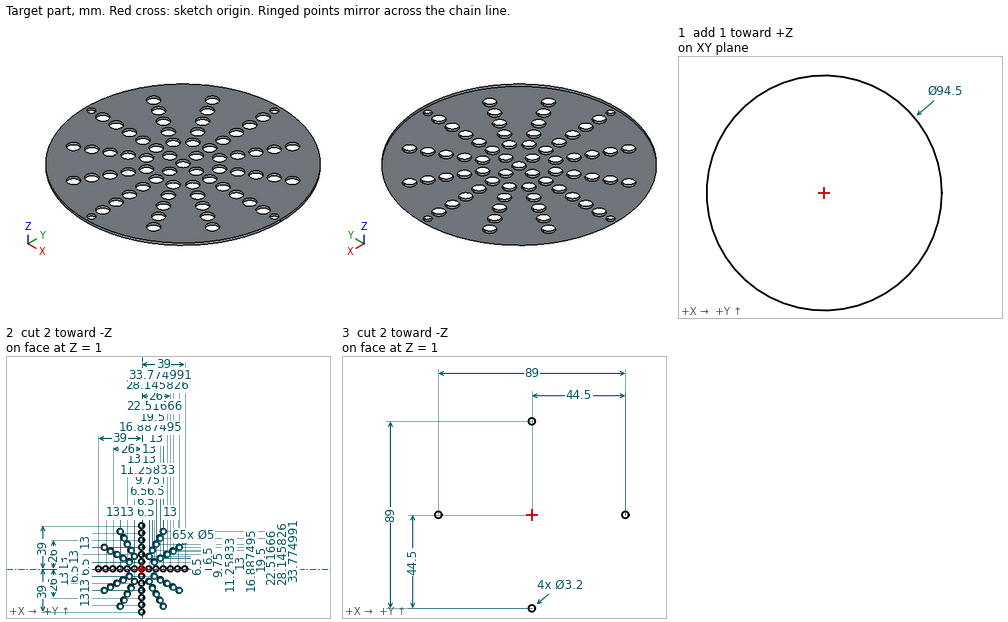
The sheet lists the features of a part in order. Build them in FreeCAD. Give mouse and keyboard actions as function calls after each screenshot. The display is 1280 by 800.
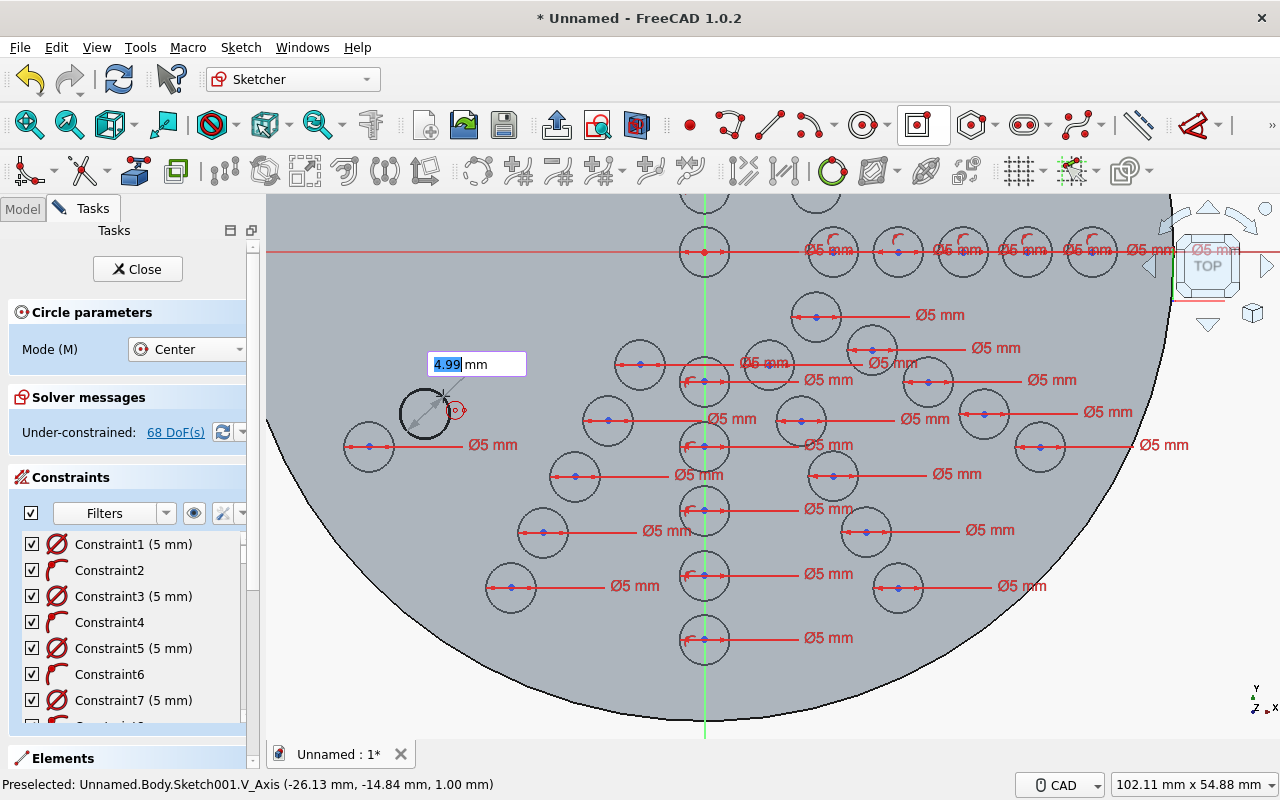
text(5)
key(Return)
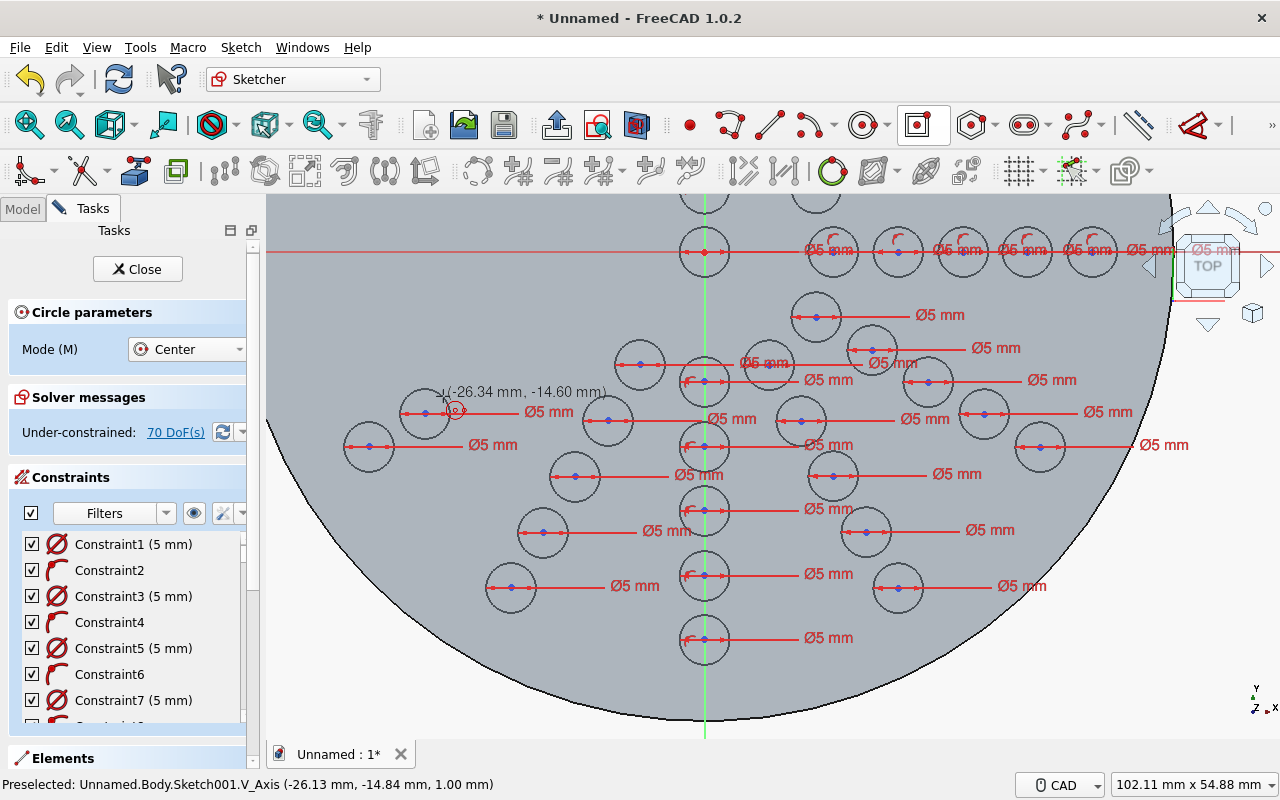
click(481, 381)
move(499, 364)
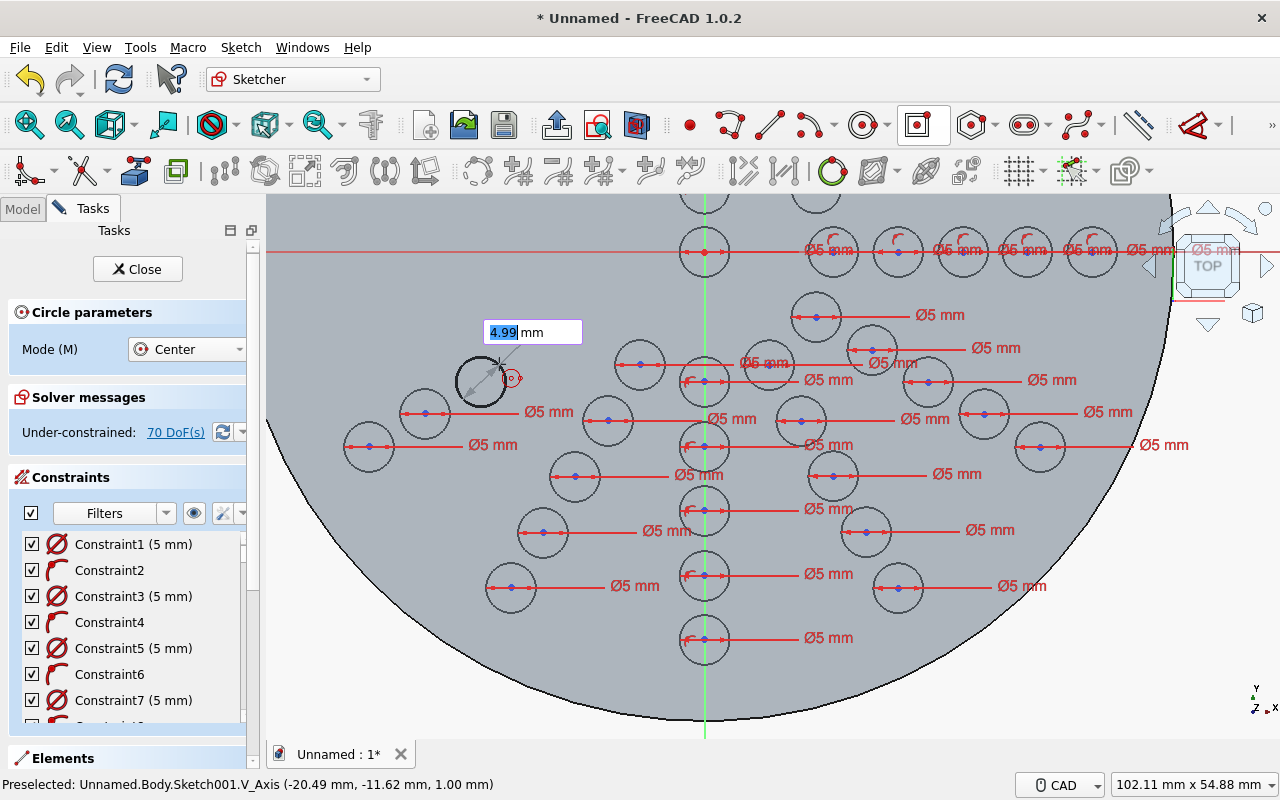
text(5)
key(Return)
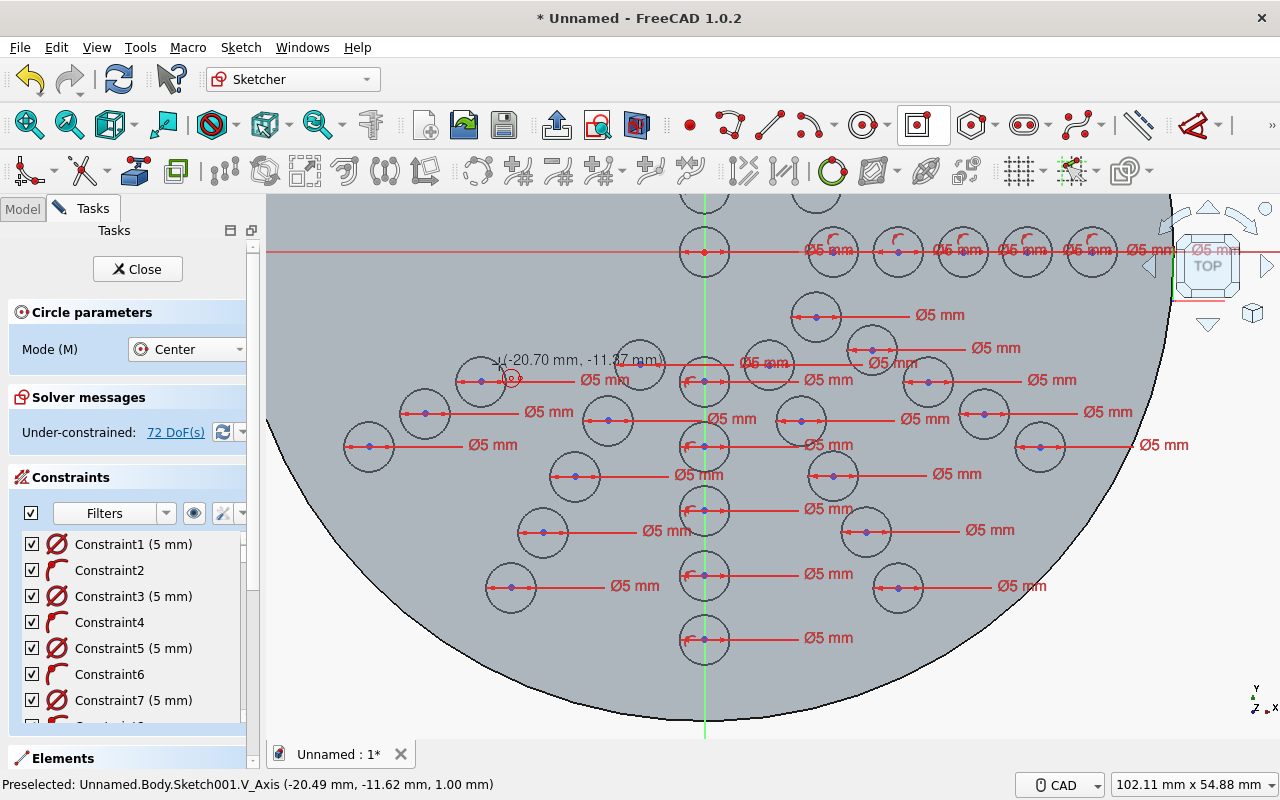
click(537, 349)
move(554, 331)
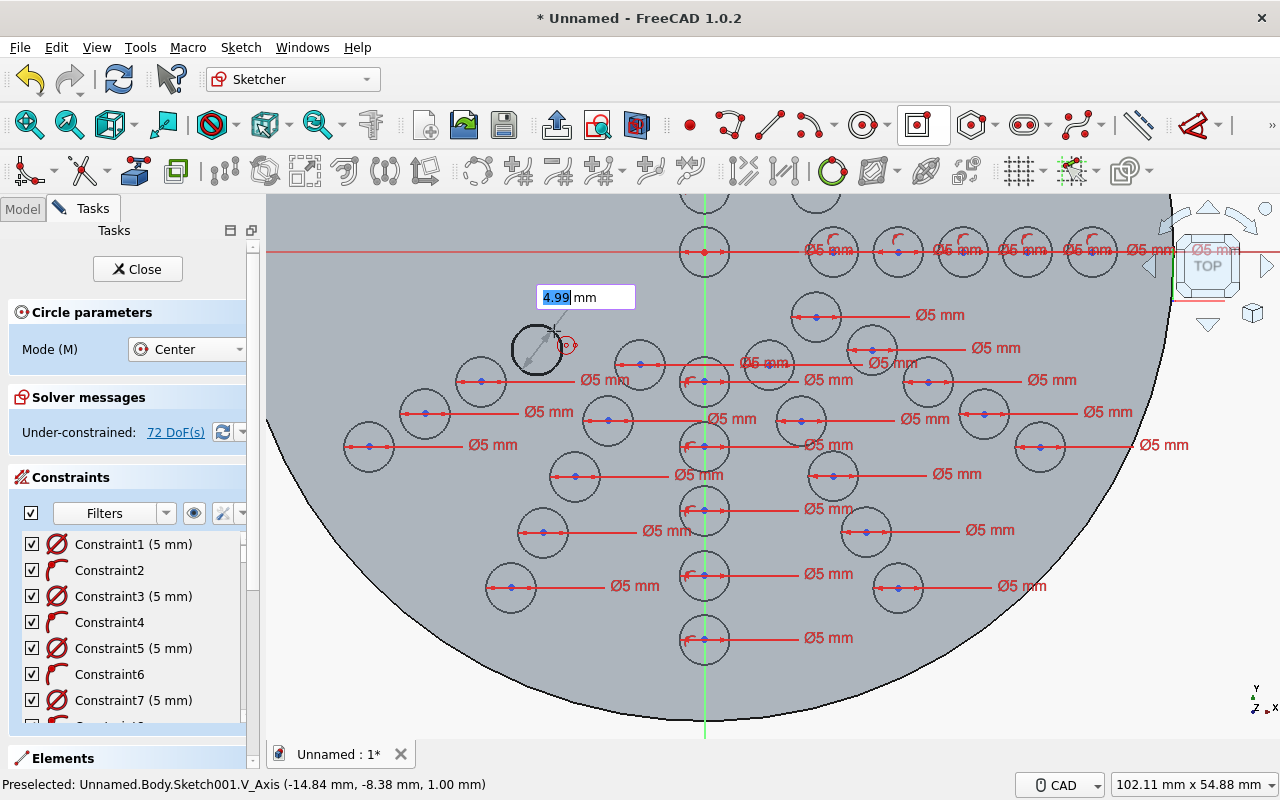
text(5)
key(Return)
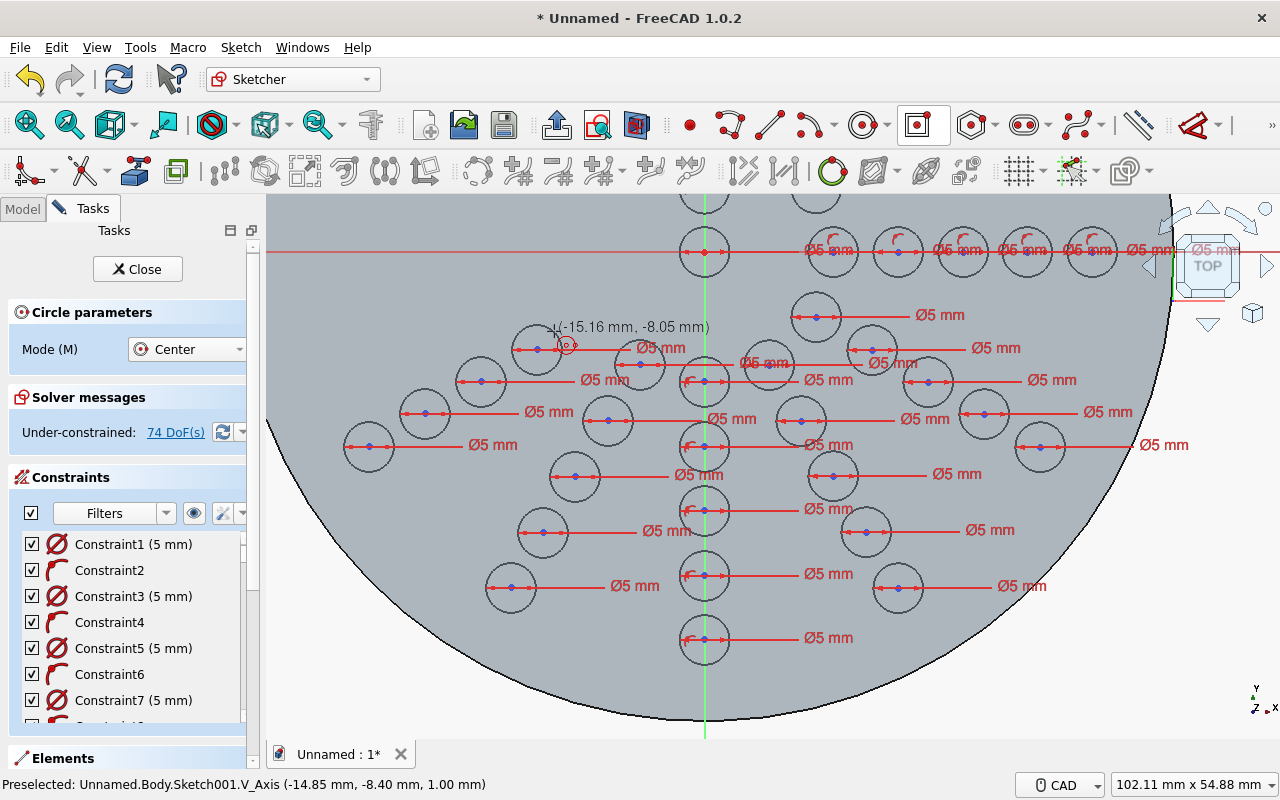
click(593, 317)
move(610, 299)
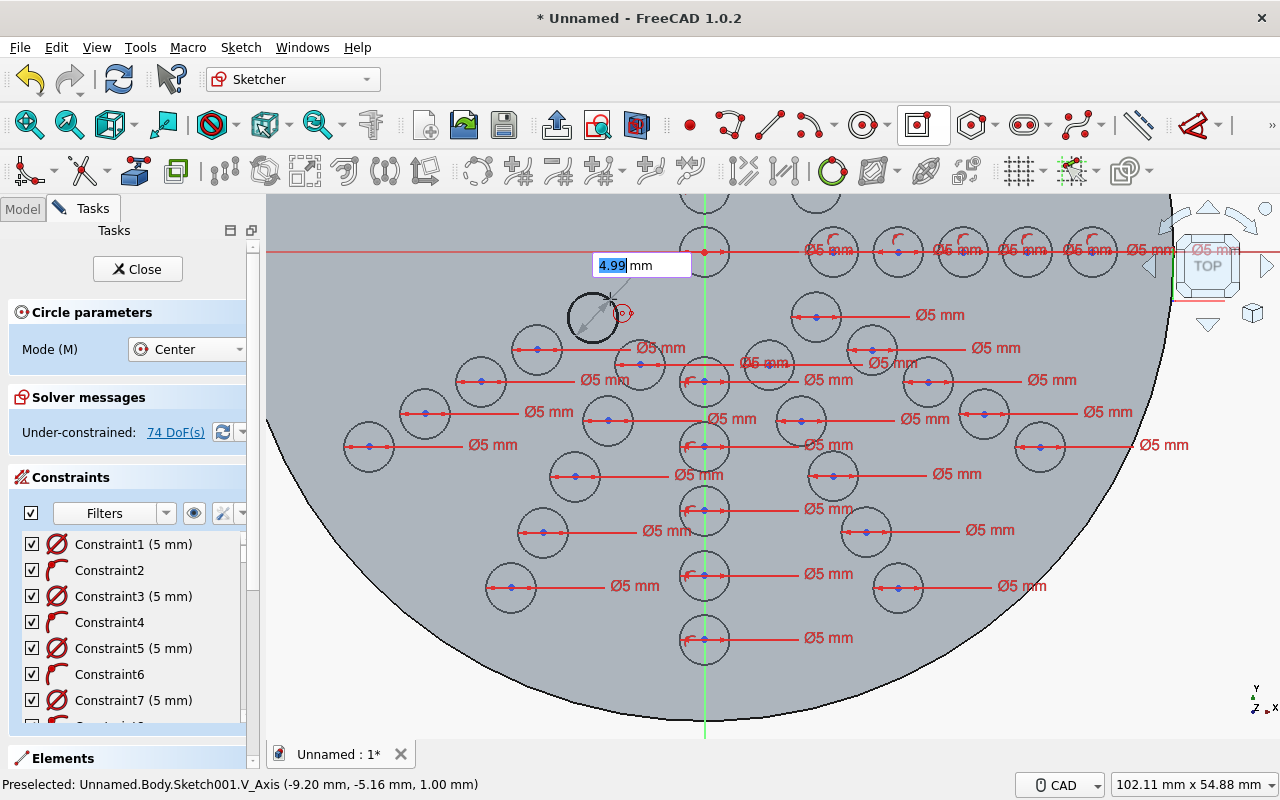
text(5)
key(Return)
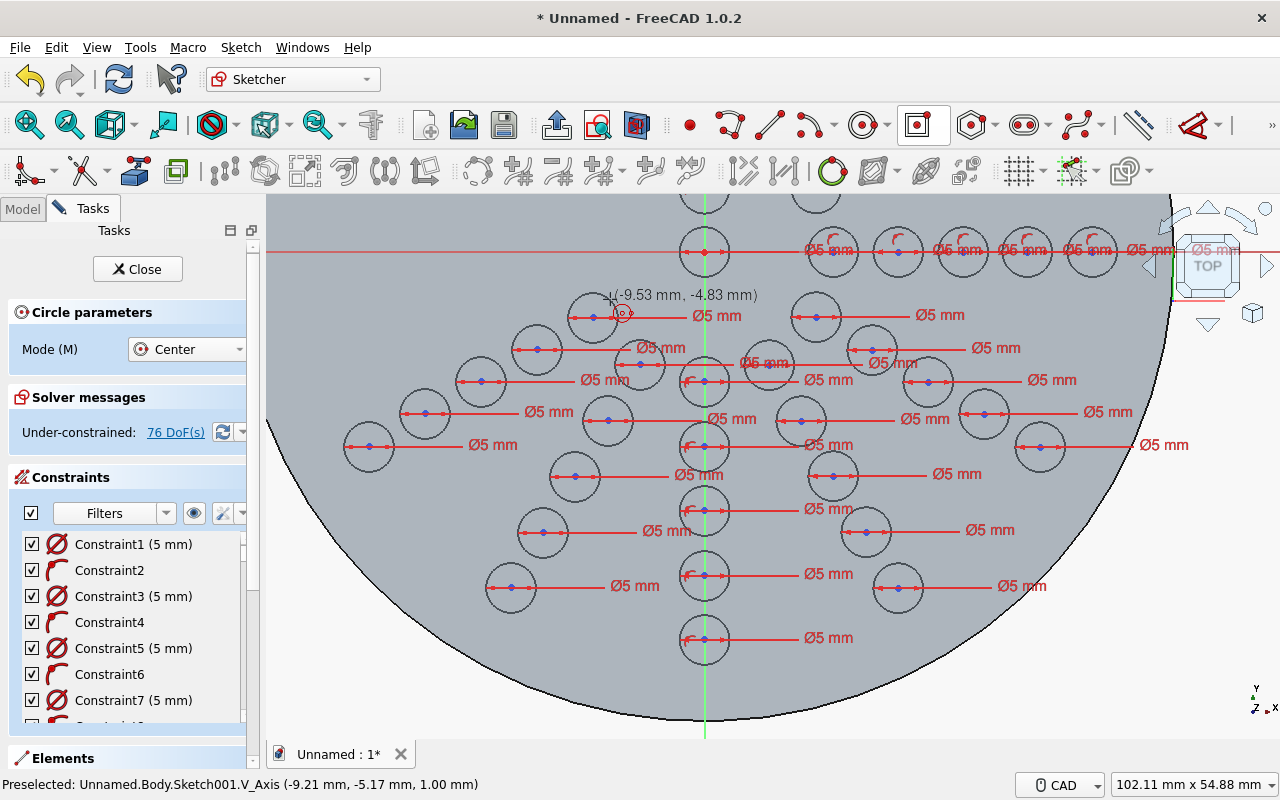
click(317, 252)
move(335, 234)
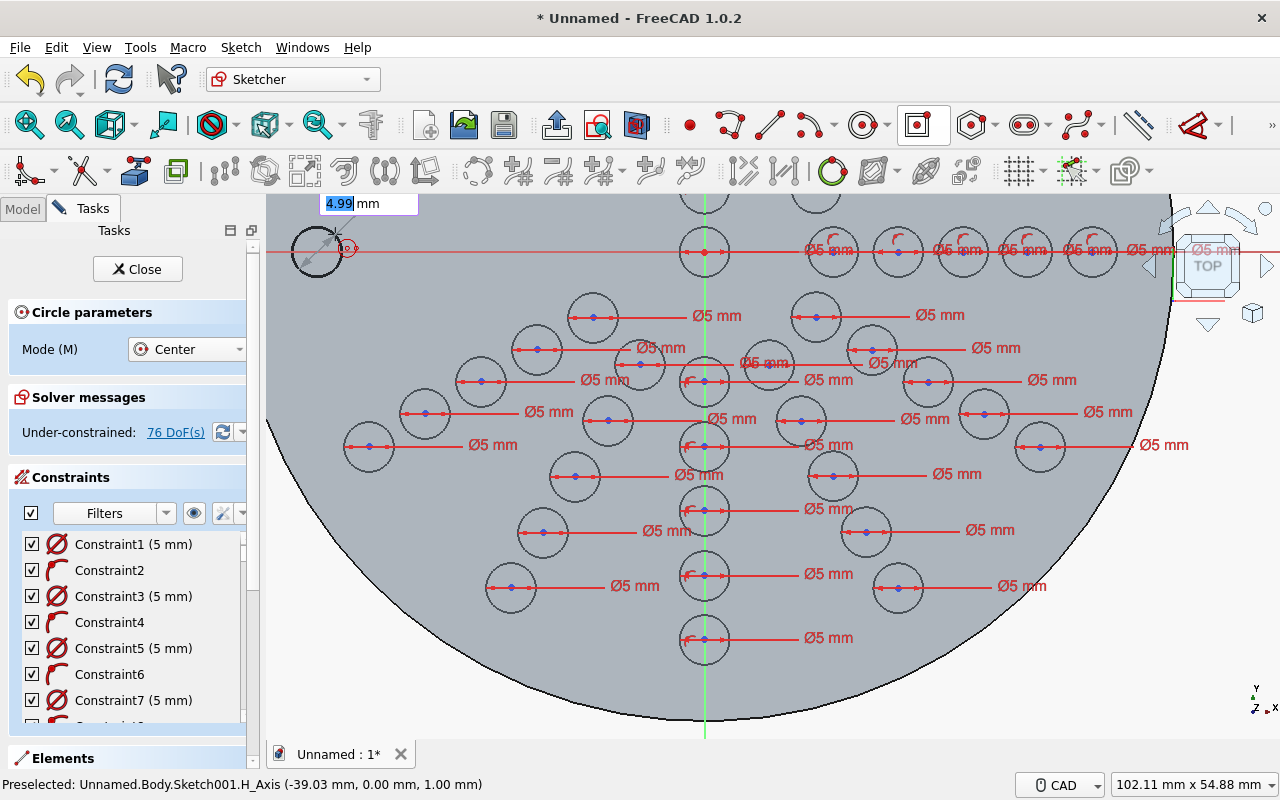
text(5)
key(Return)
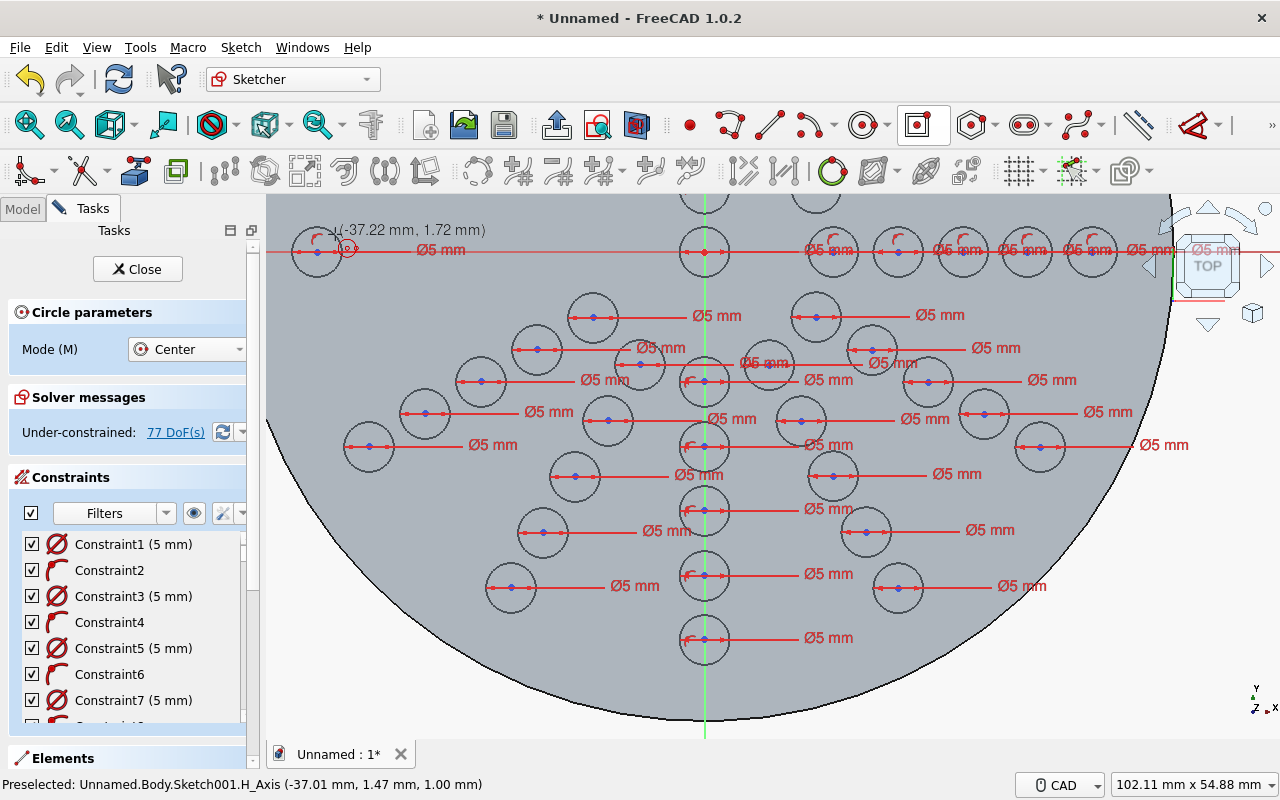
click(382, 252)
move(399, 234)